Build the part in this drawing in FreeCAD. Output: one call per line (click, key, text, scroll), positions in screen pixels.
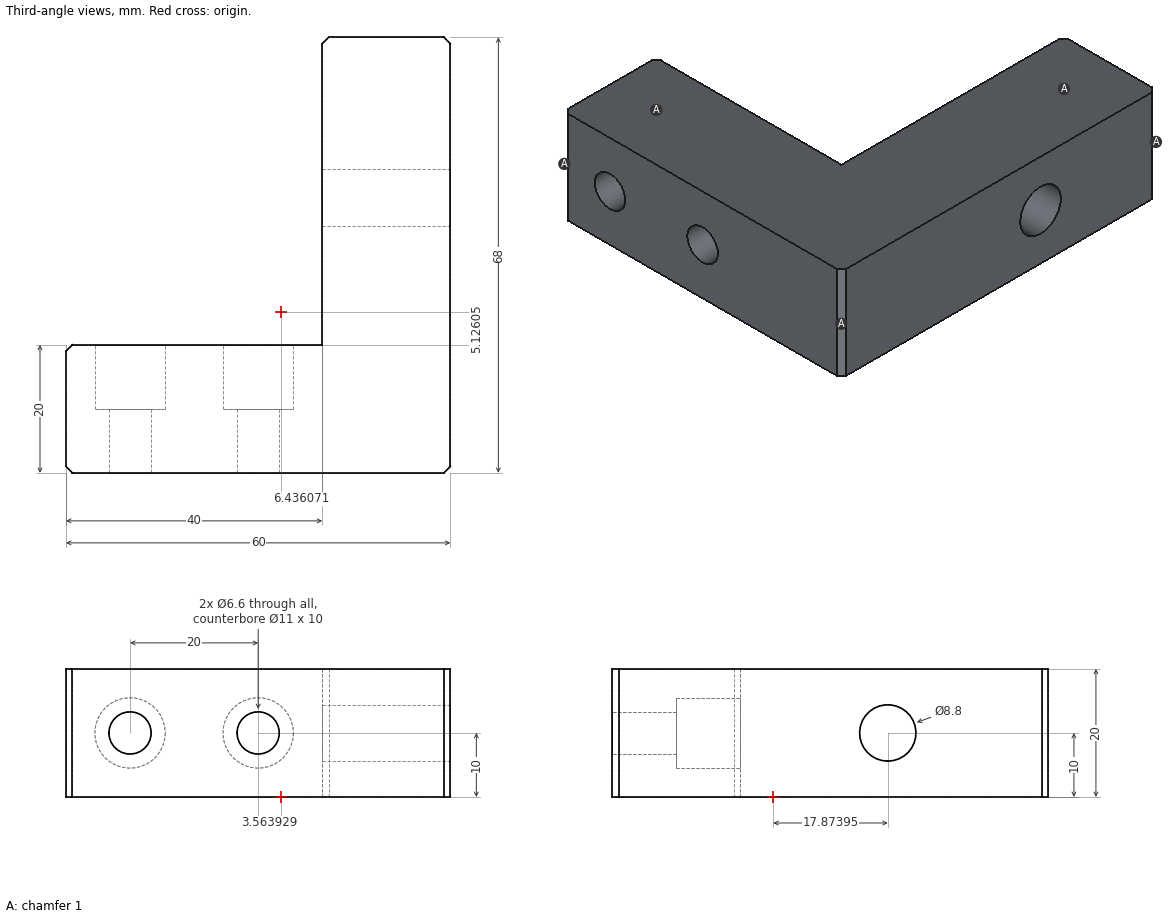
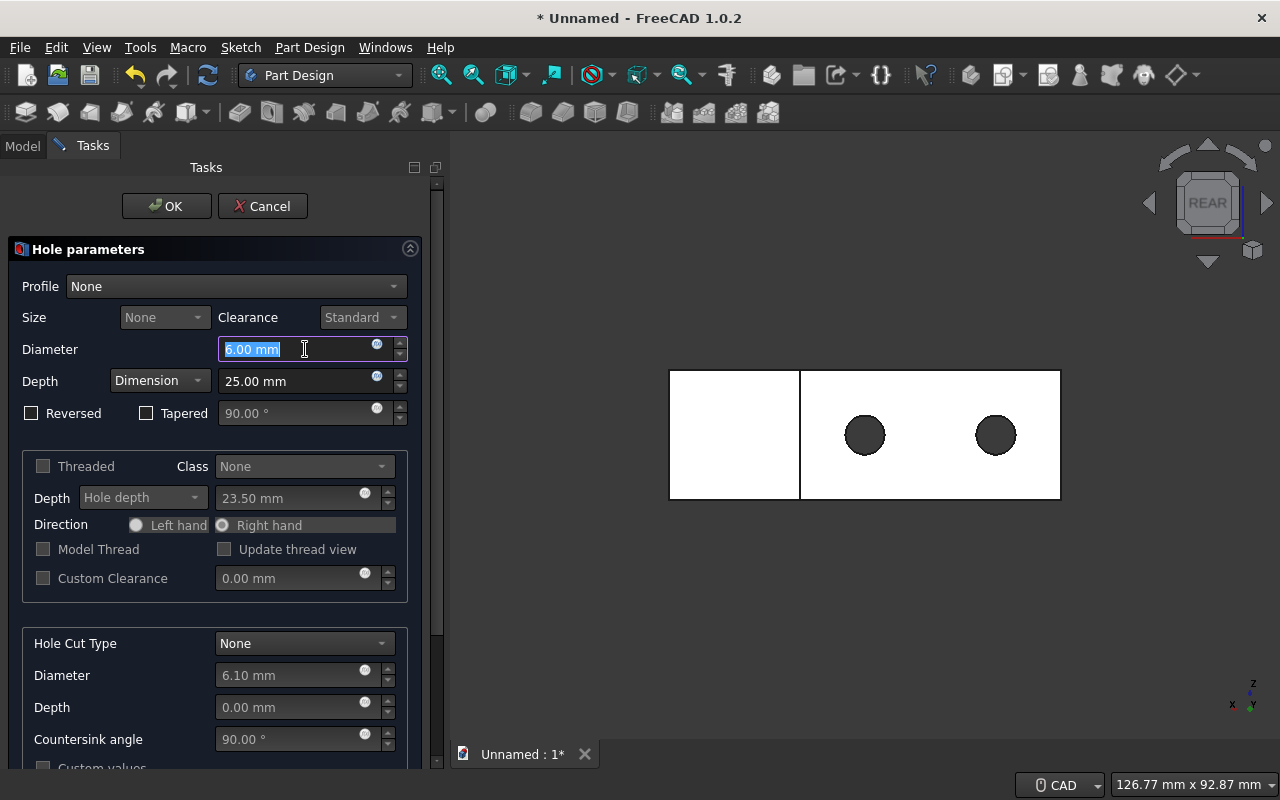
text(6.6)
key(Tab)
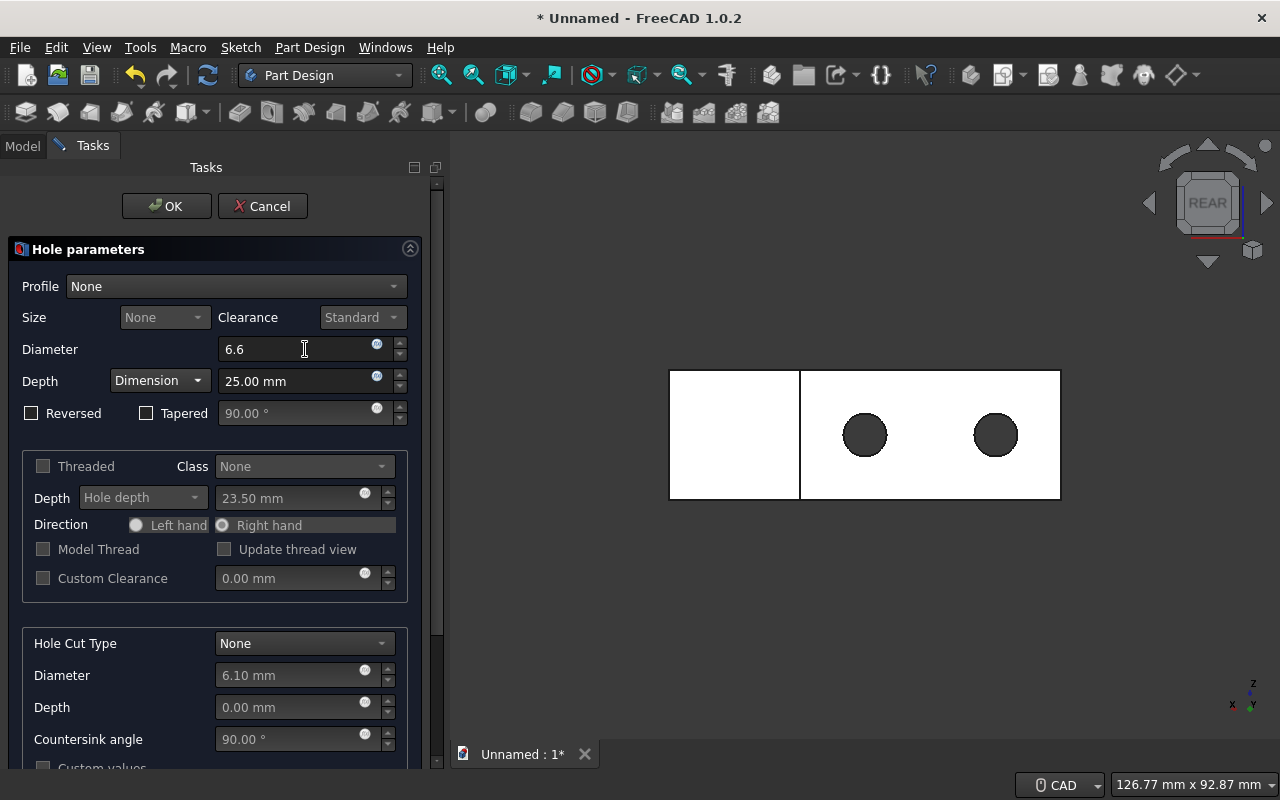
click(161, 380)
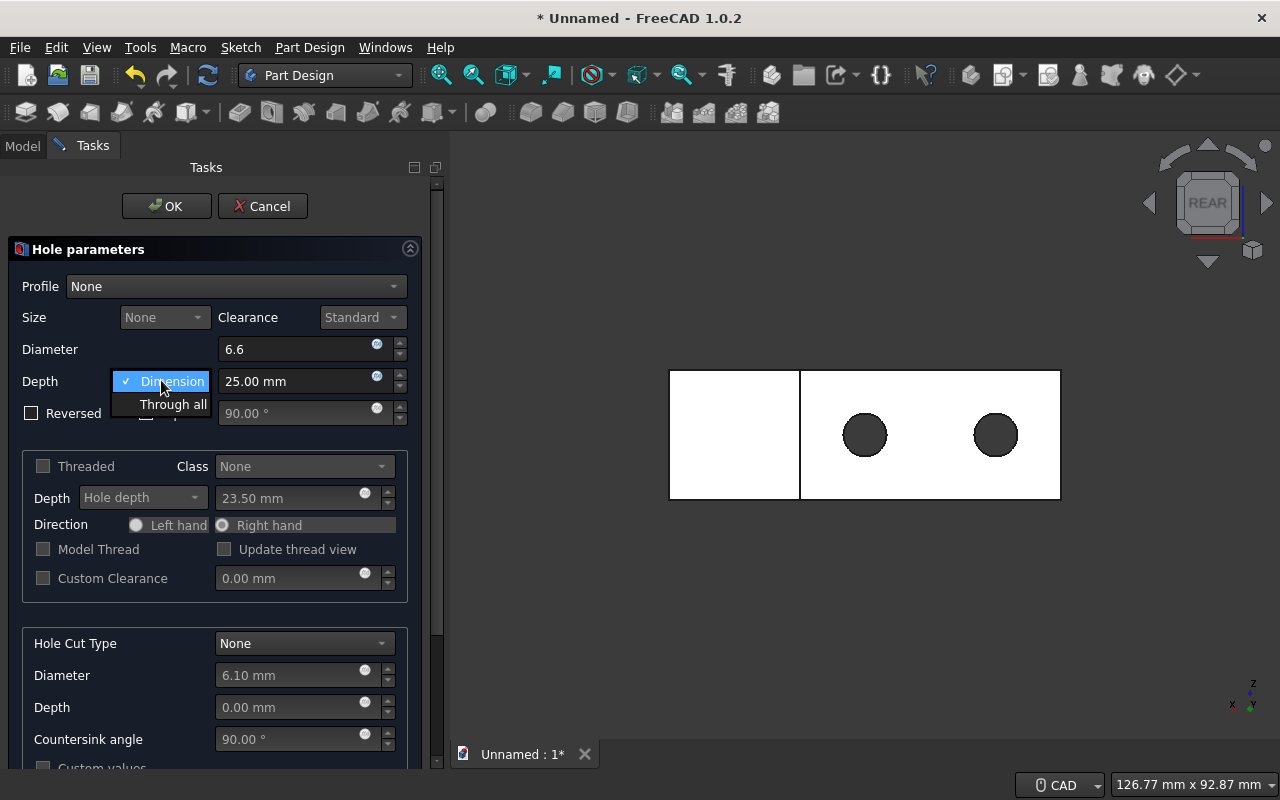
click(160, 404)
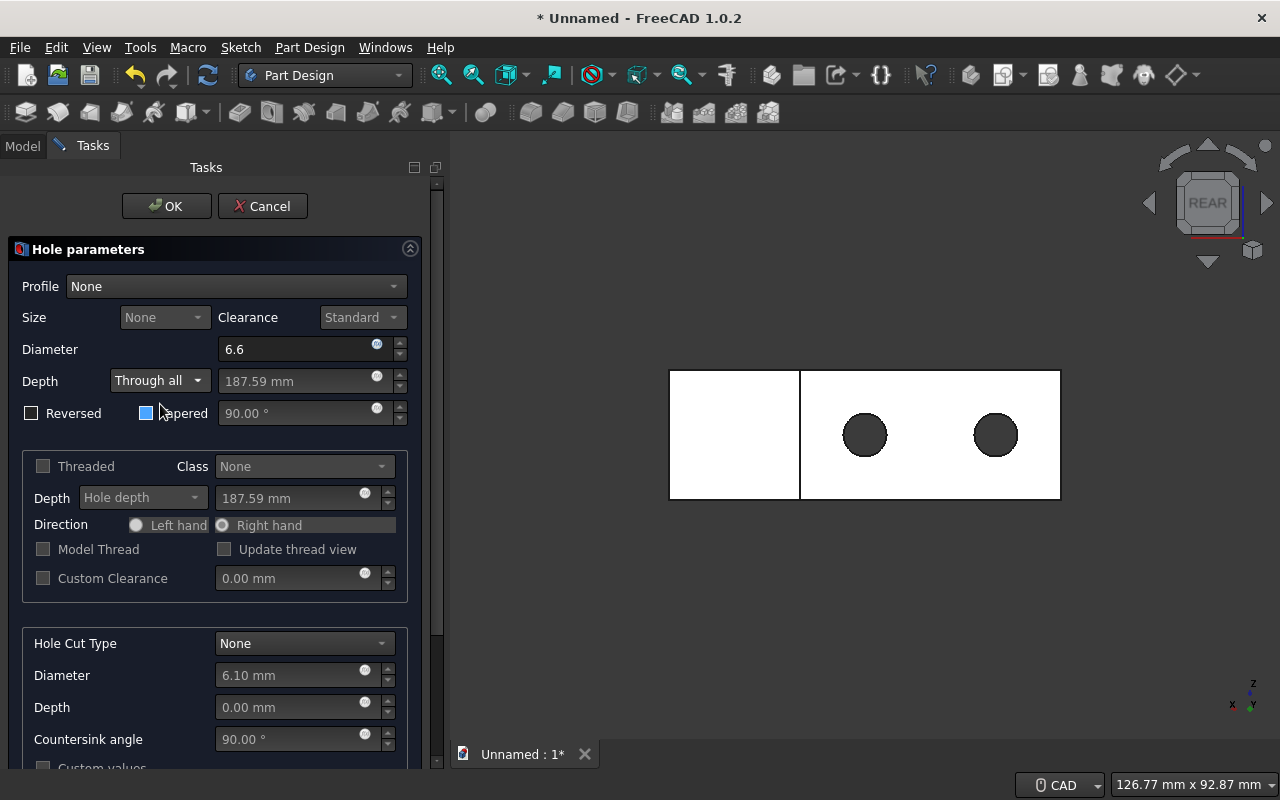
click(306, 644)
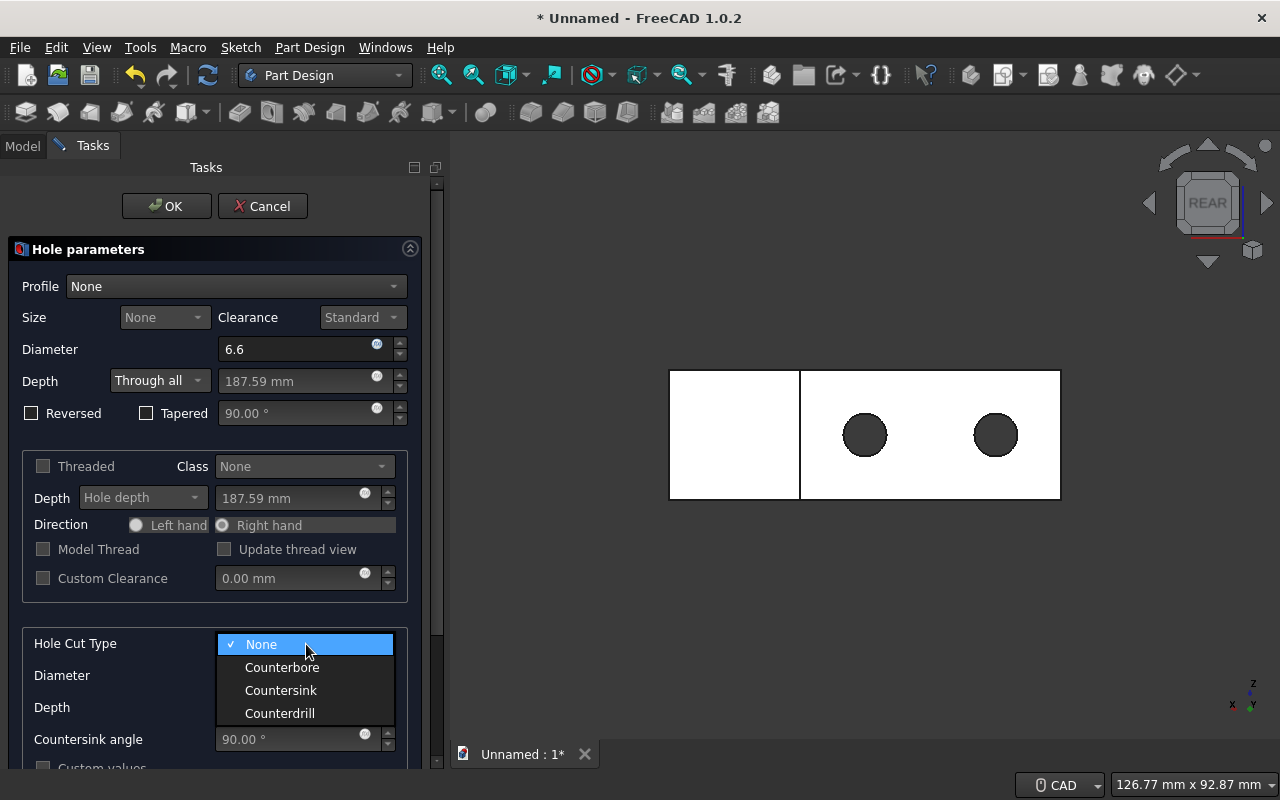
click(304, 668)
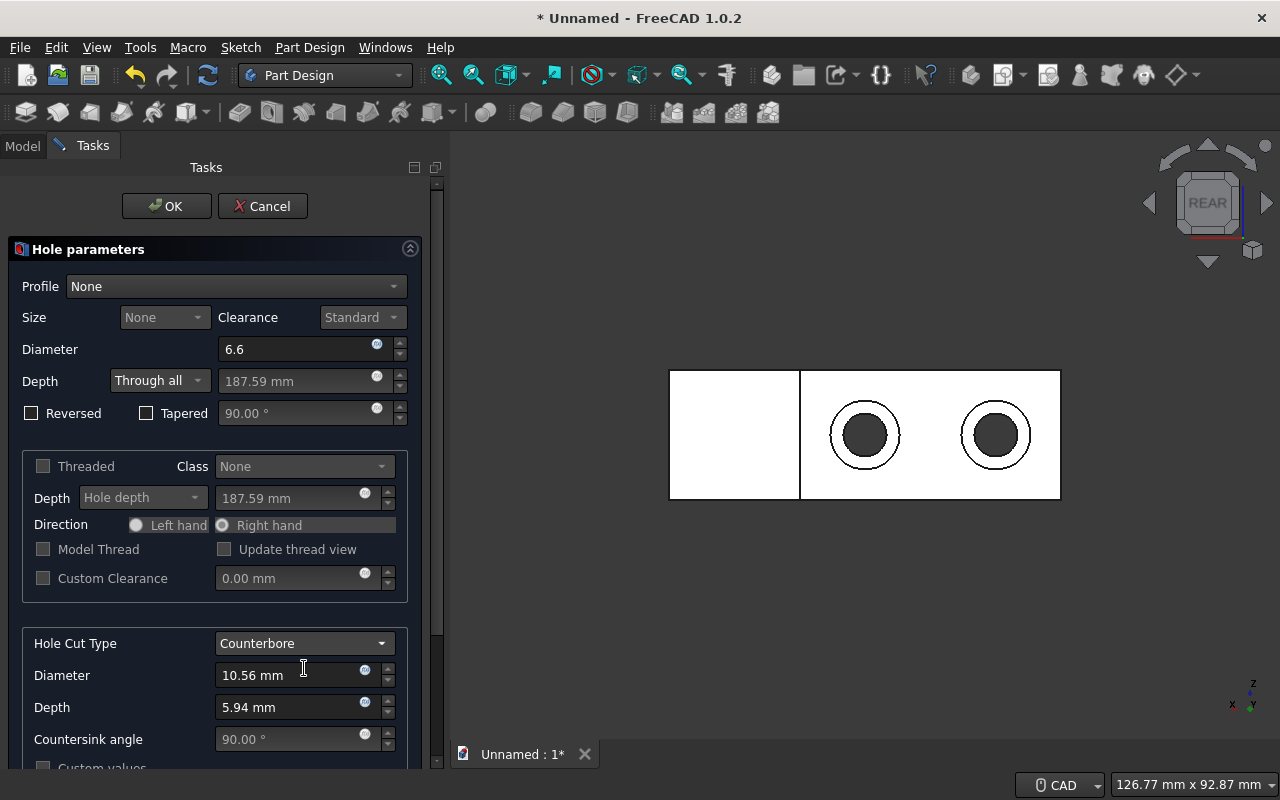
triple_click(298, 675)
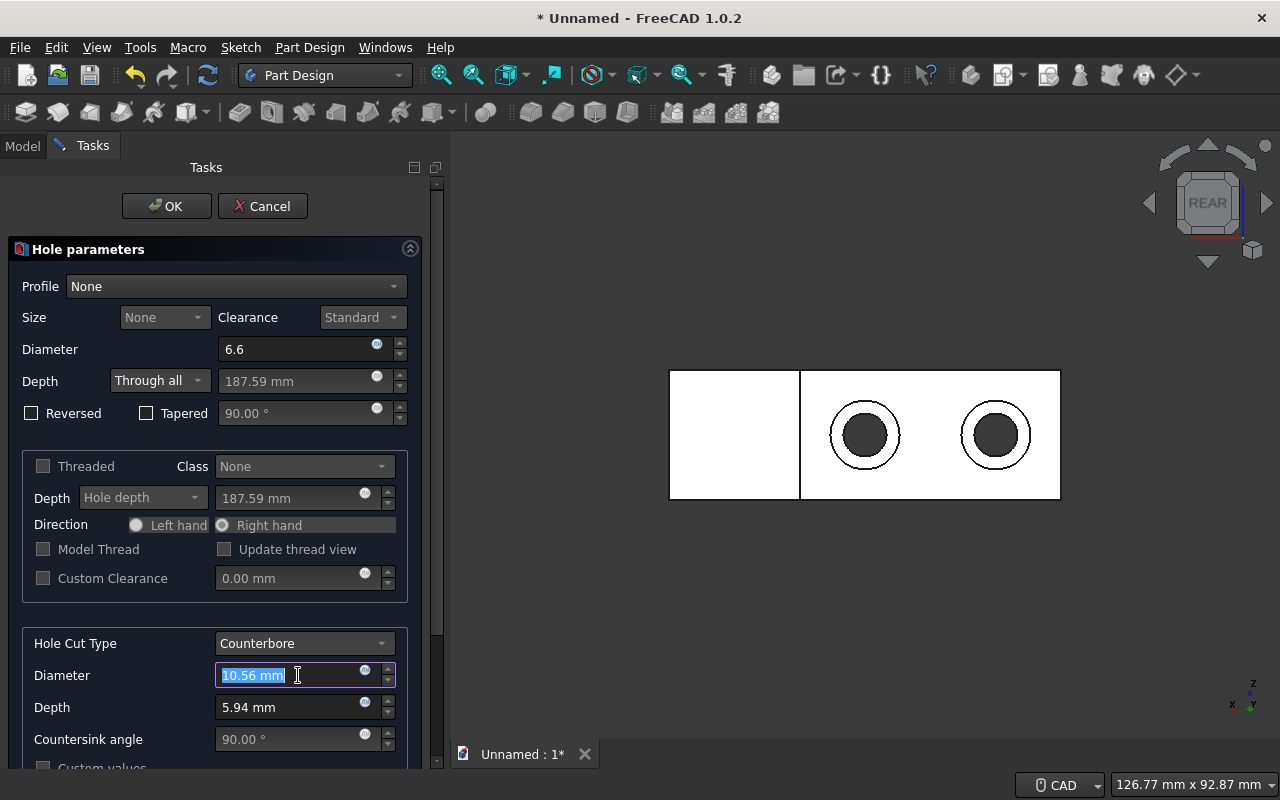
text(11)
key(Tab)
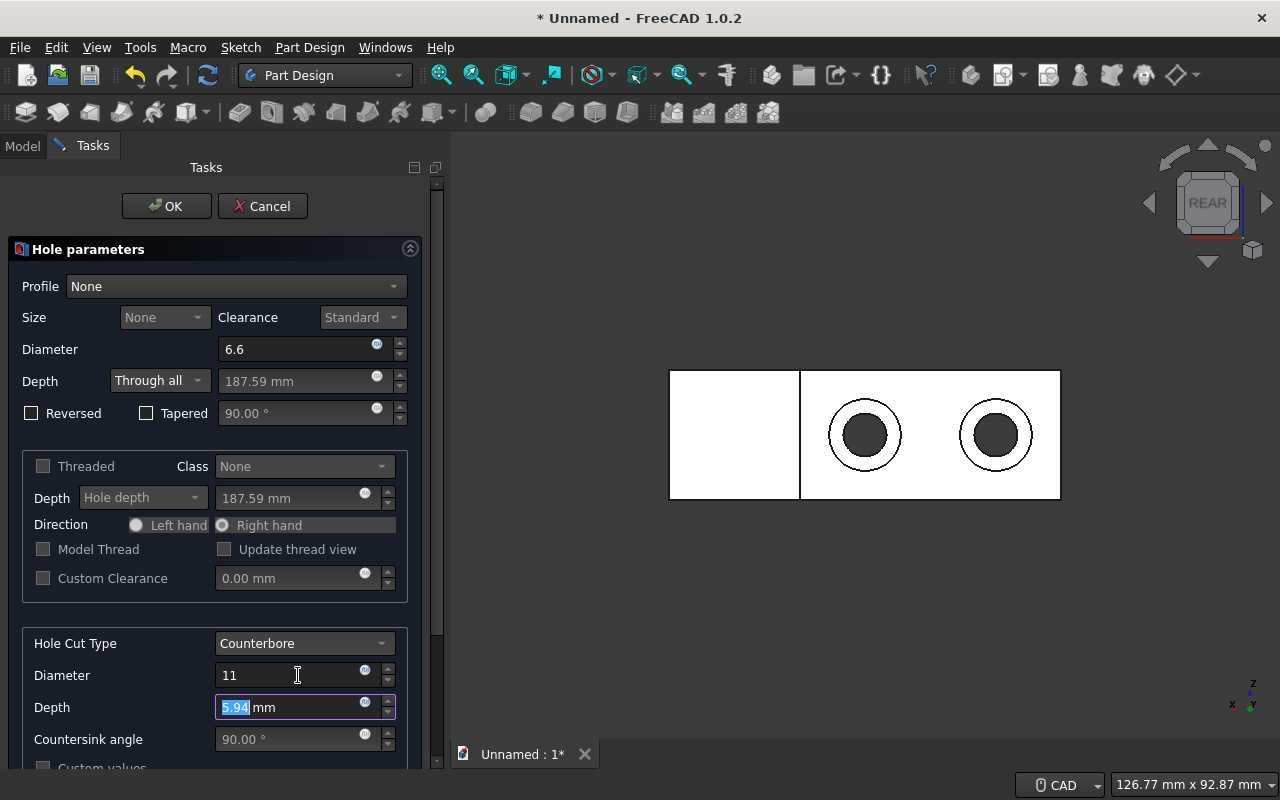
text(10)
key(Tab)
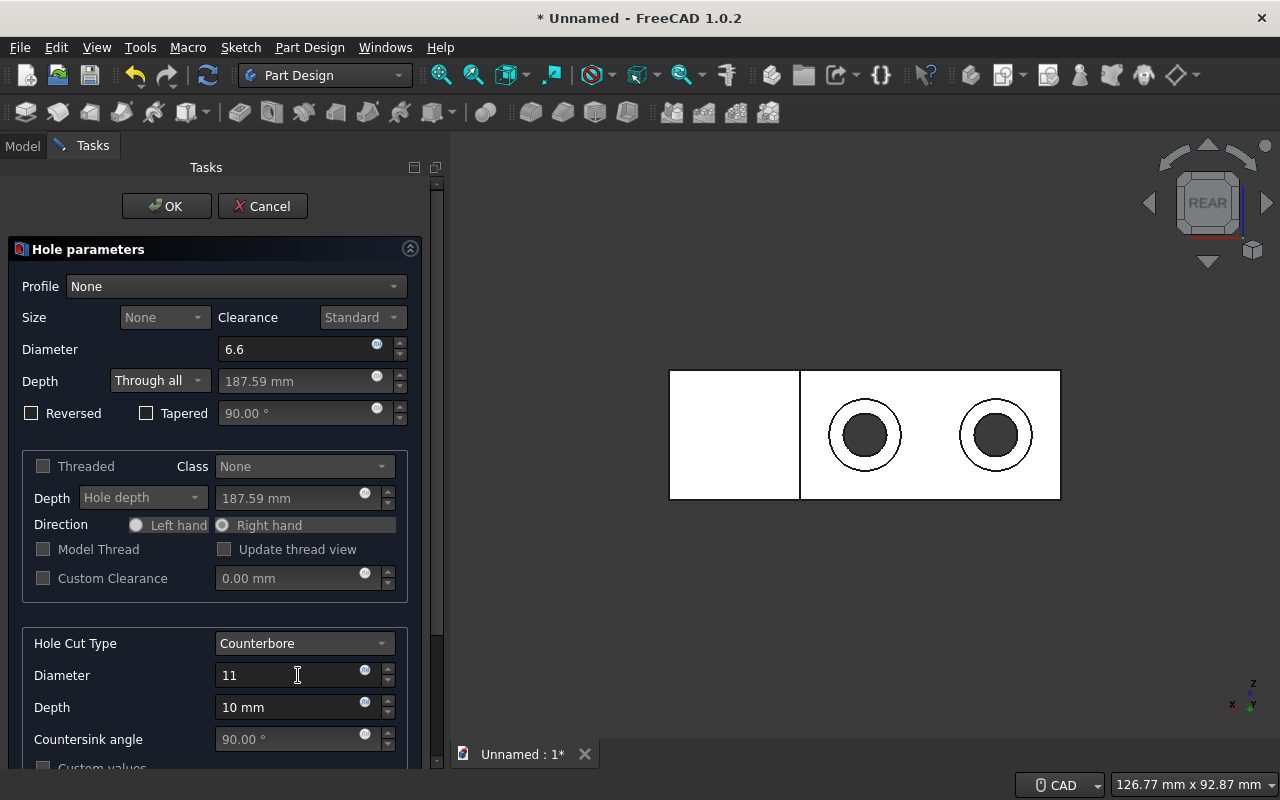
click(167, 206)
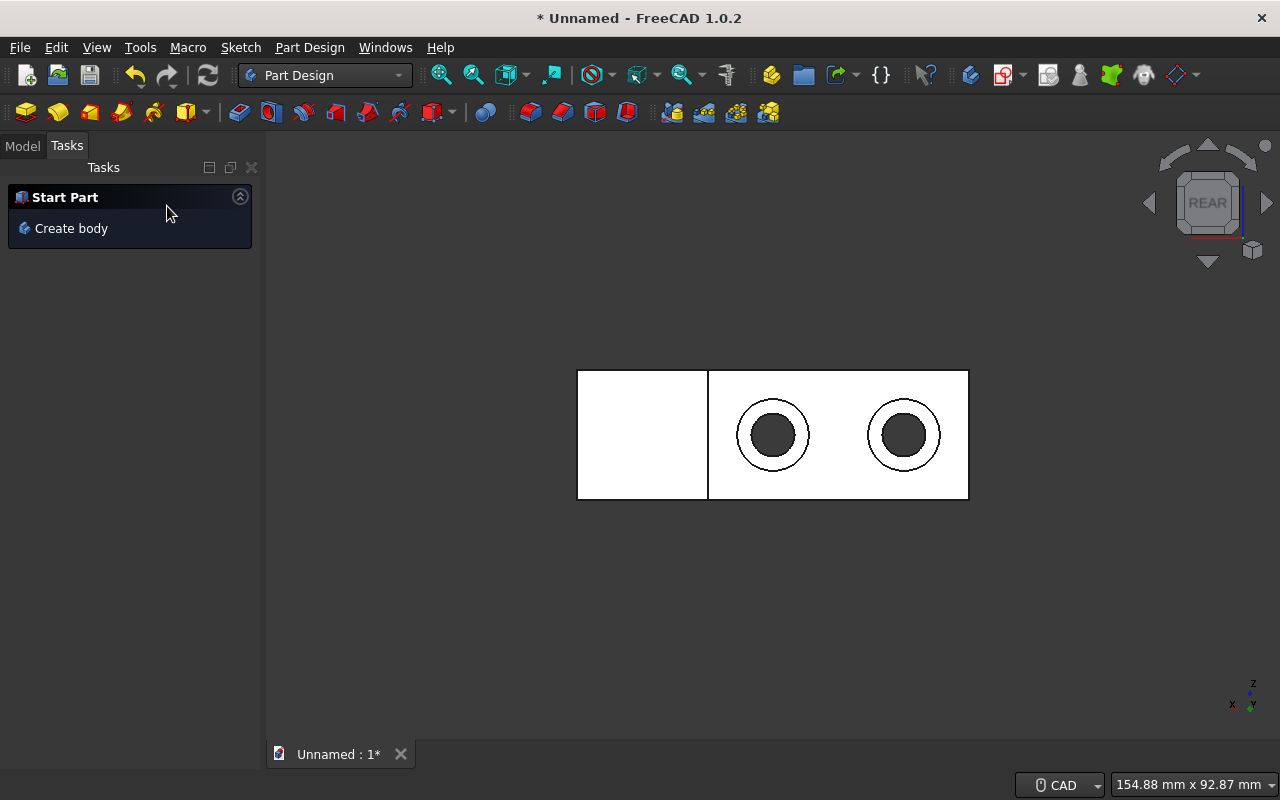
click(442, 76)